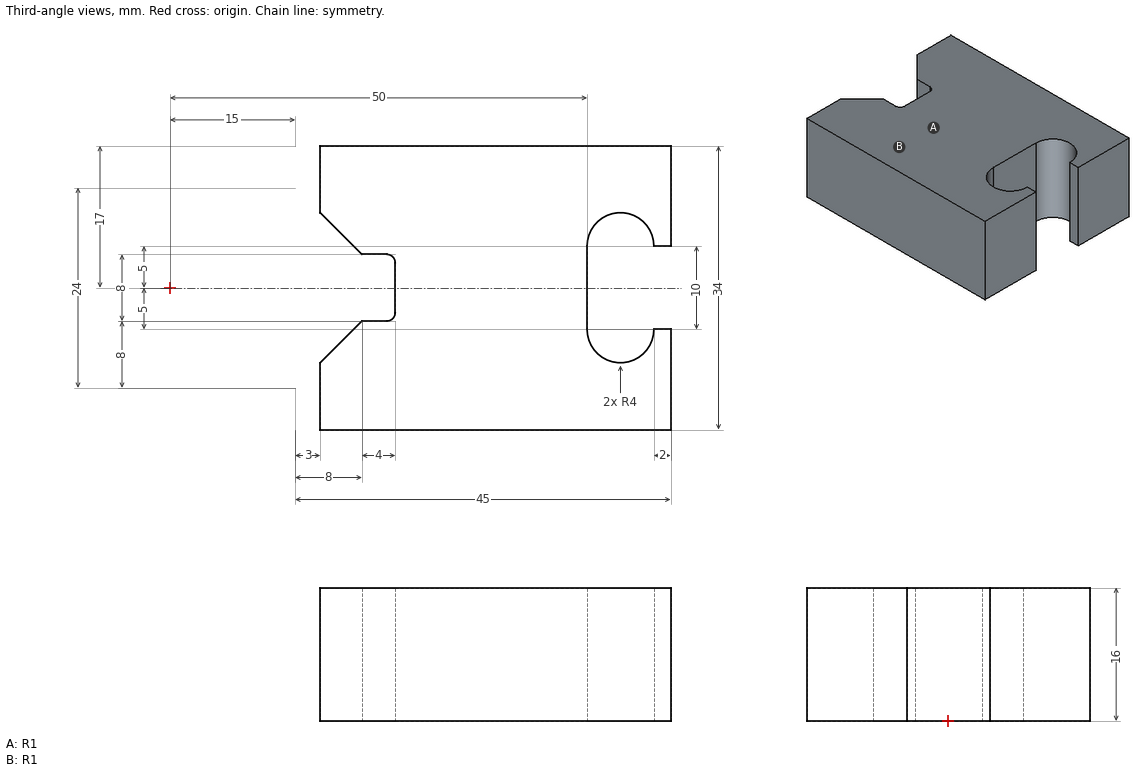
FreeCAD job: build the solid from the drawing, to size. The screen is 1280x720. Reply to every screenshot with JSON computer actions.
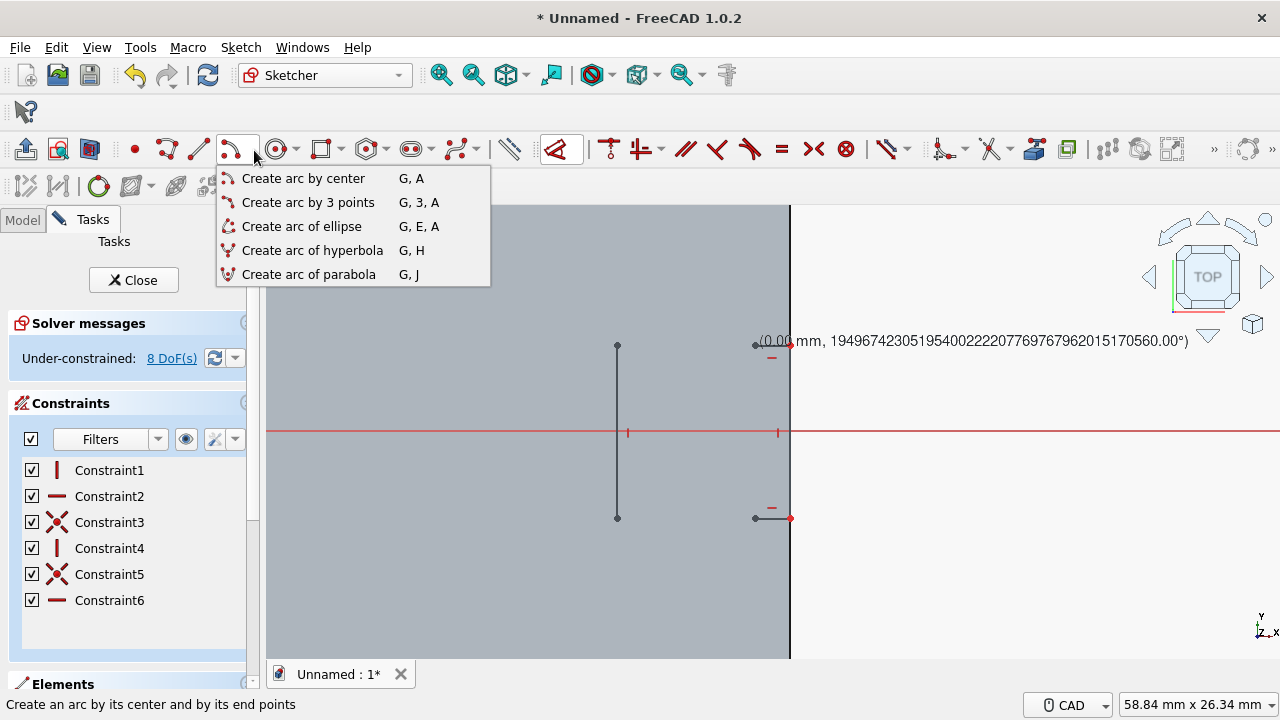
{"action": "left_click", "coordinate": [354, 202]}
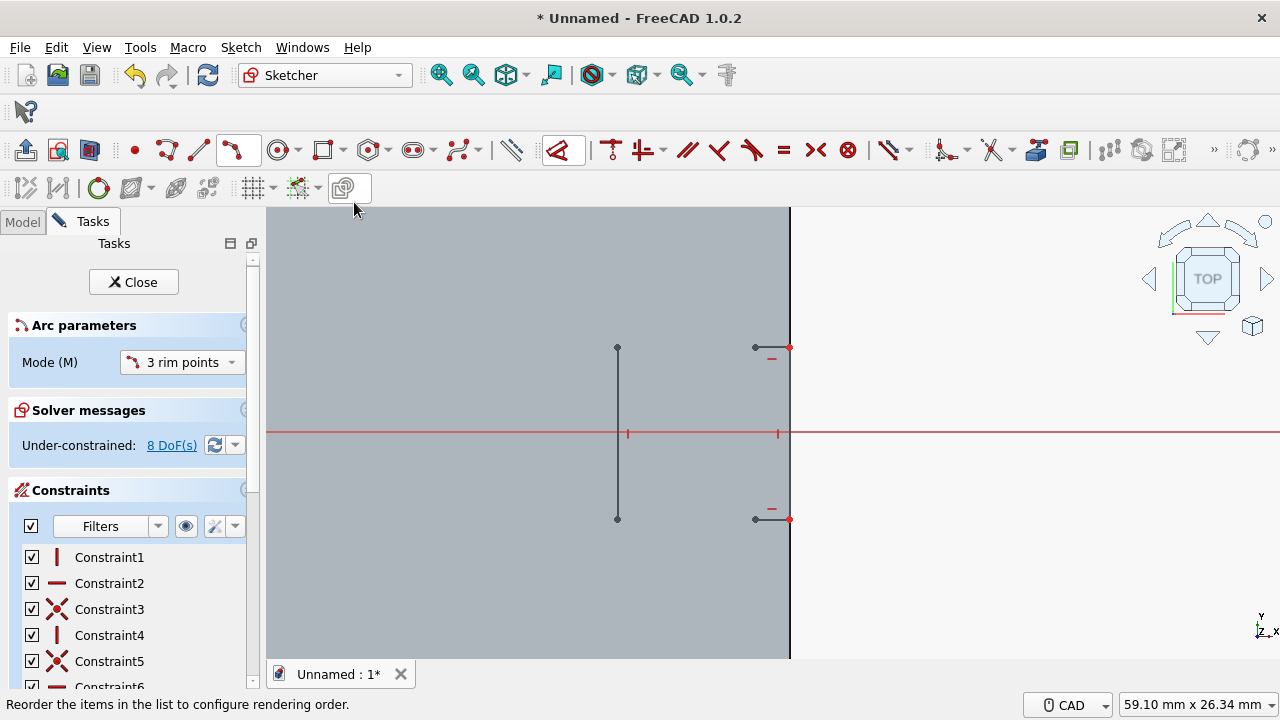
{"action": "left_click", "coordinate": [618, 520]}
{"action": "left_click", "coordinate": [755, 520]}
{"action": "left_click", "coordinate": [687, 587]}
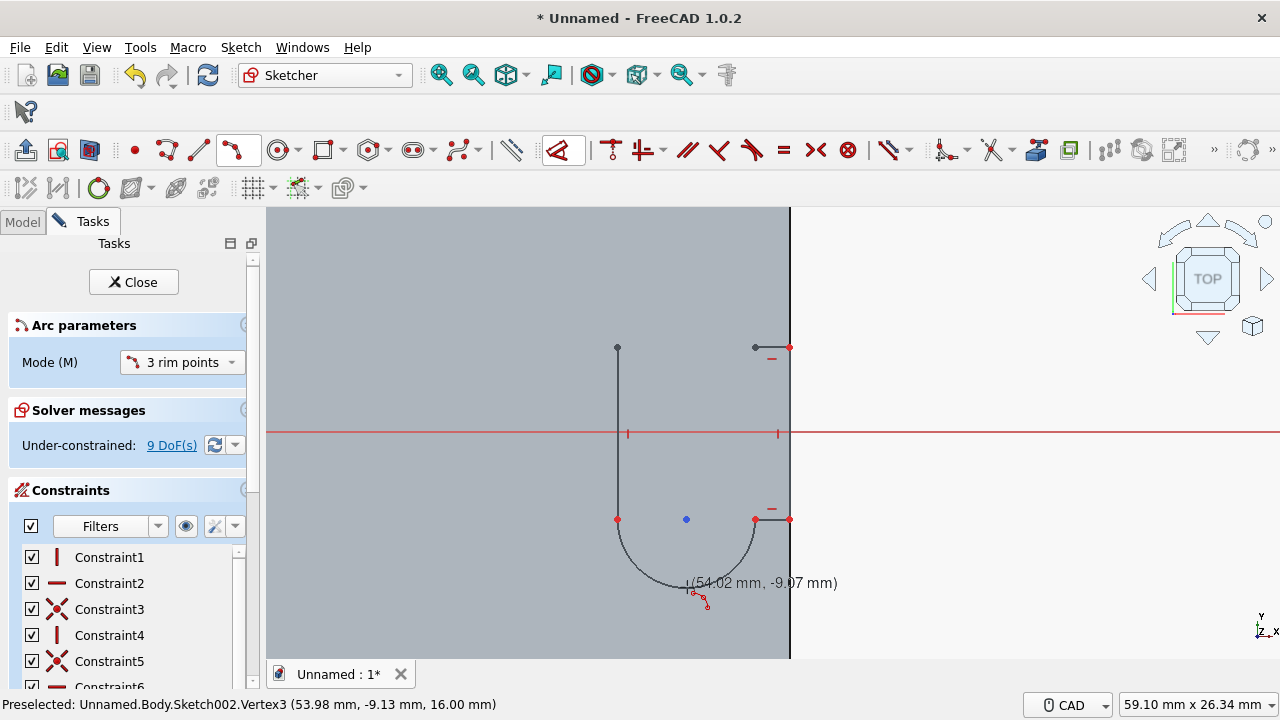
{"action": "left_click", "coordinate": [755, 347]}
{"action": "left_click", "coordinate": [618, 347]}
{"action": "left_click", "coordinate": [687, 278]}
{"action": "key", "text": "Escape"}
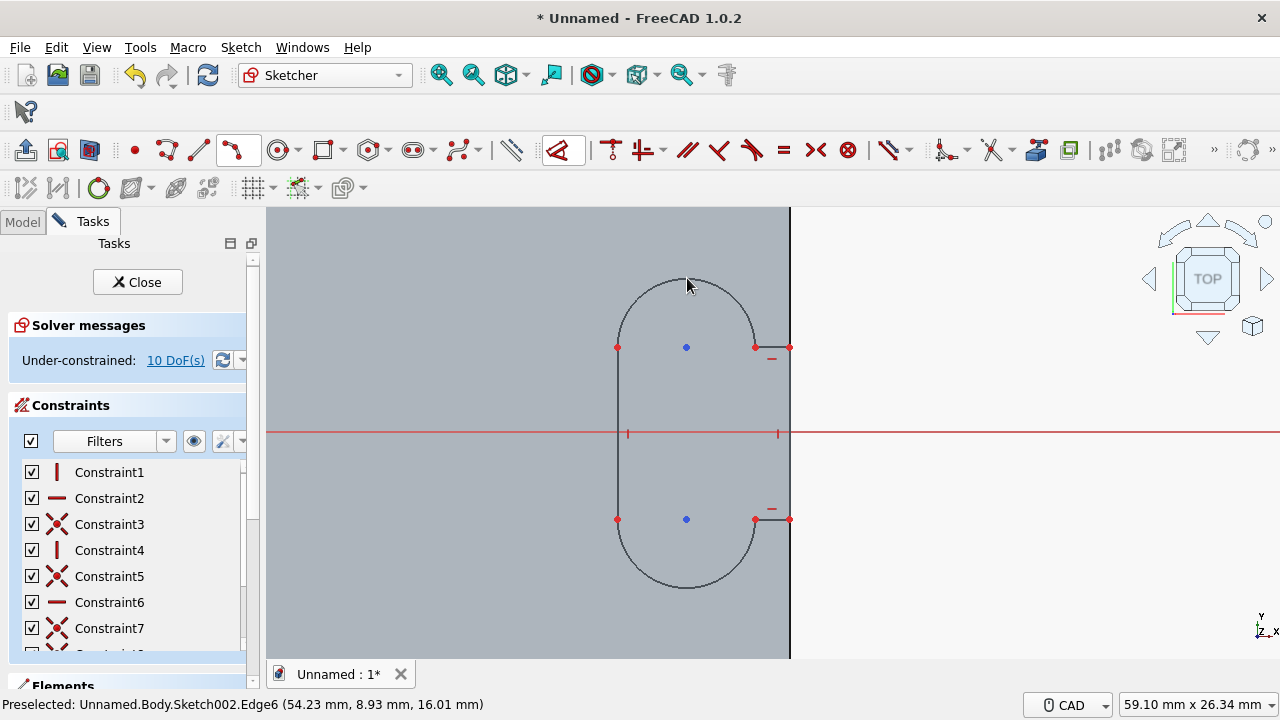
{"action": "left_click", "coordinate": [618, 399]}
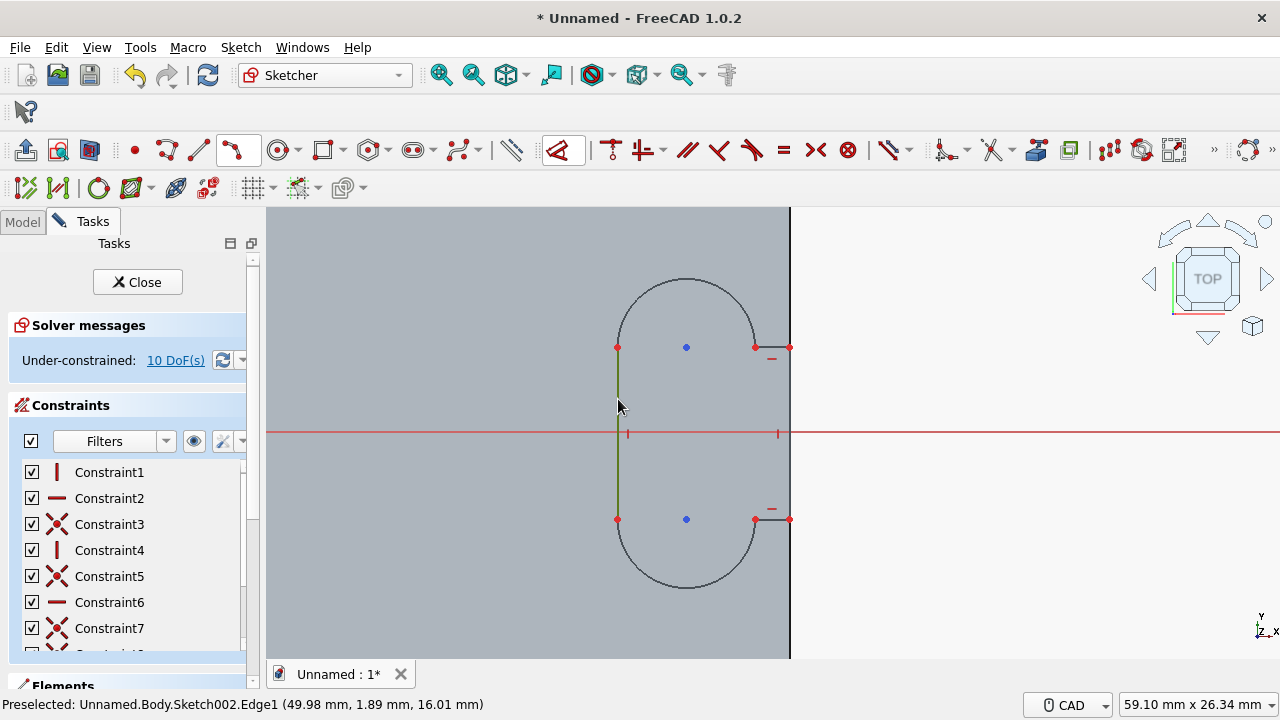
{"action": "left_click", "coordinate": [646, 575]}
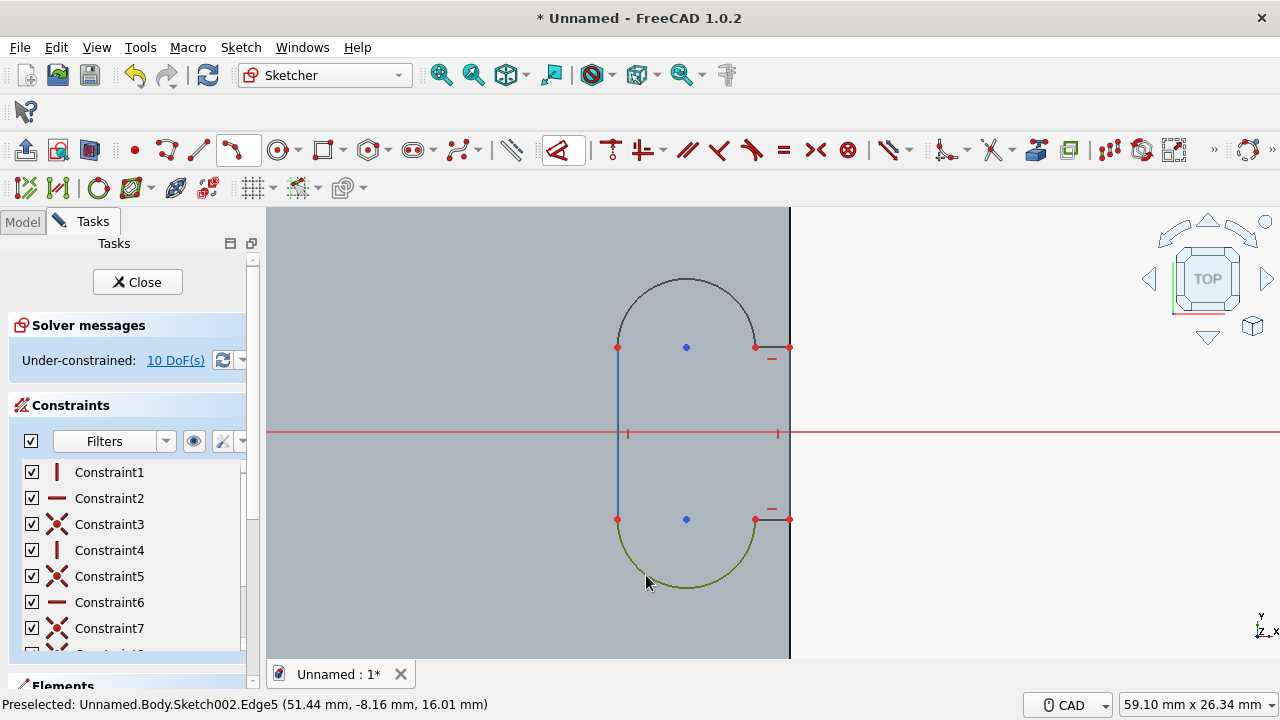
{"action": "left_click", "coordinate": [752, 150]}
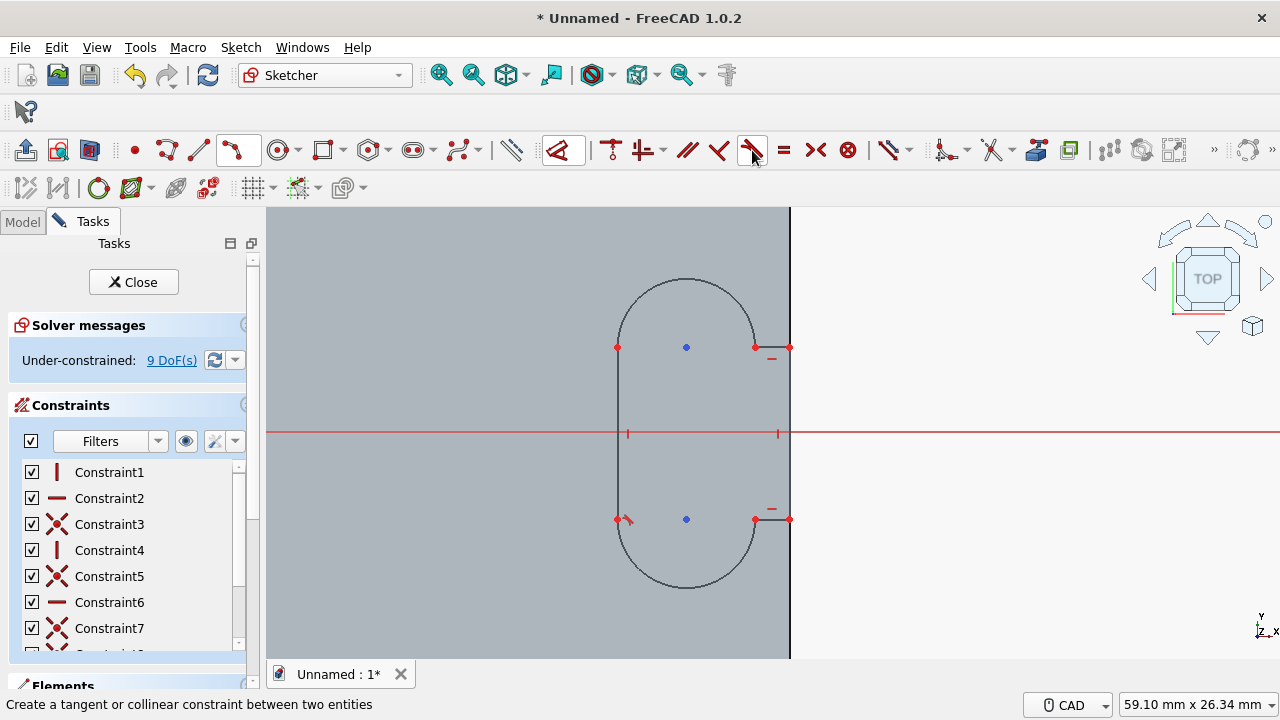
{"action": "left_click", "coordinate": [618, 399]}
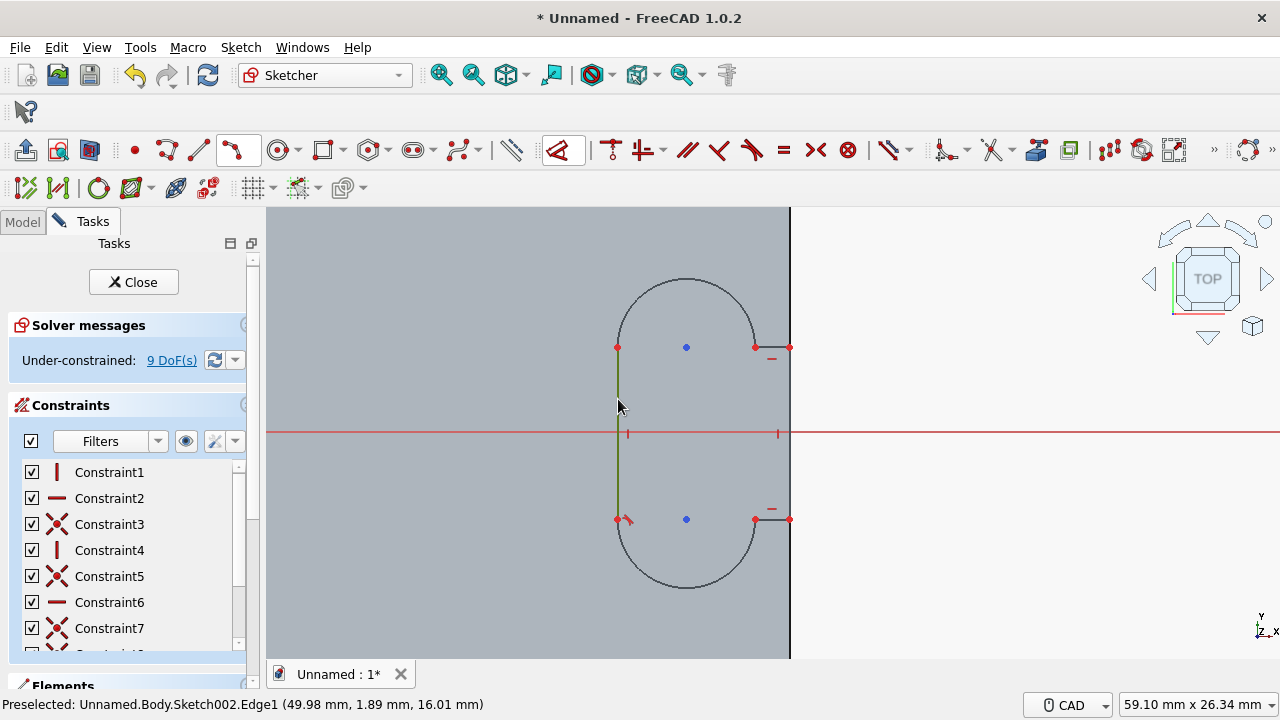
{"action": "left_click", "coordinate": [727, 292]}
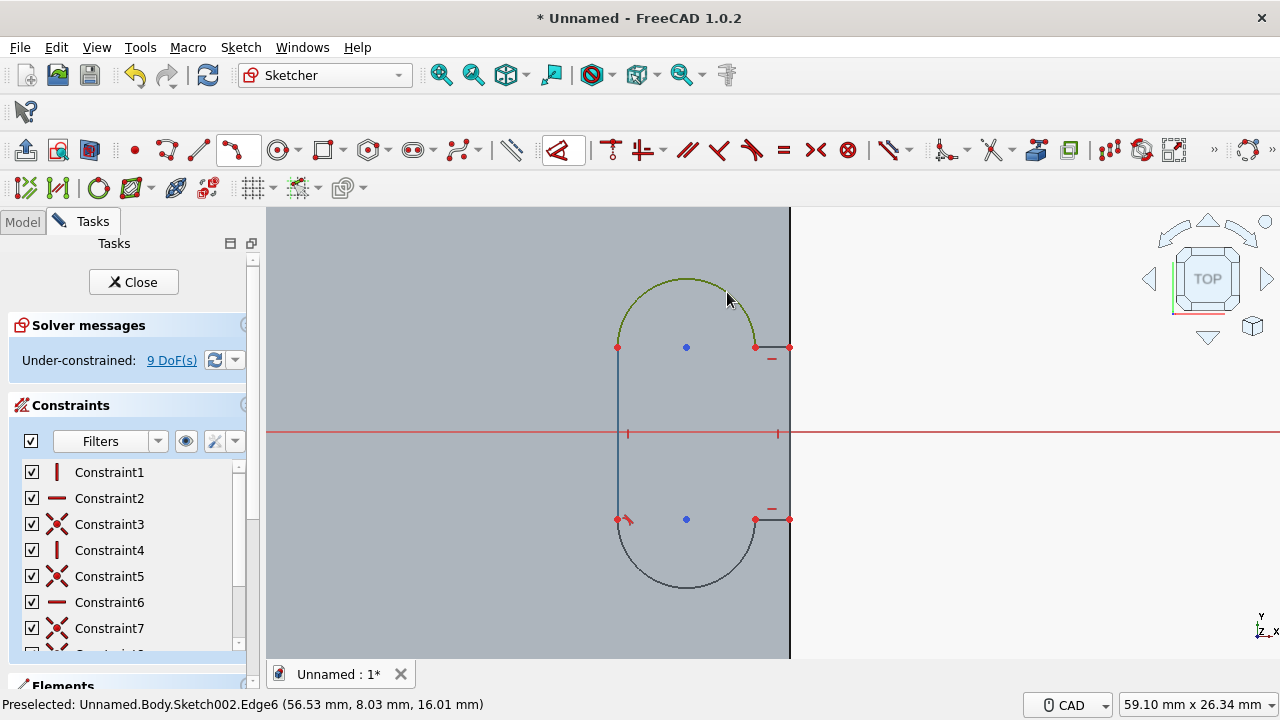
{"action": "left_click", "coordinate": [752, 150]}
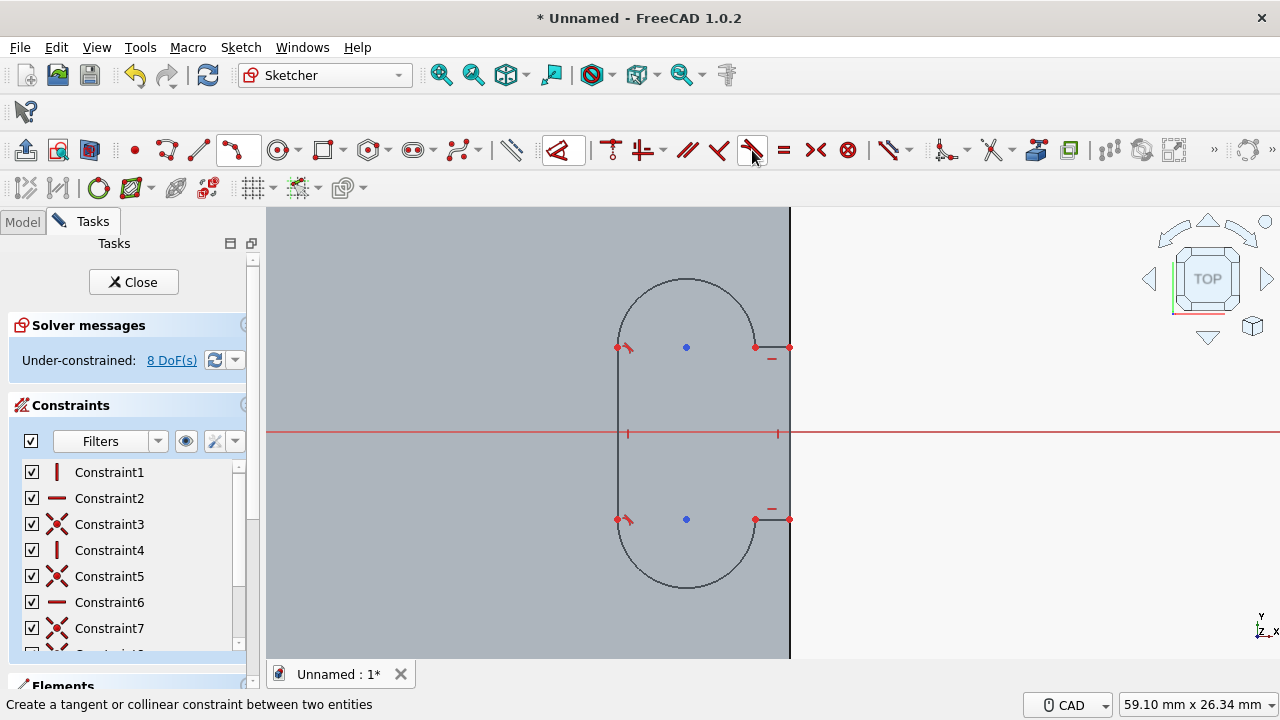
{"action": "left_click", "coordinate": [646, 575]}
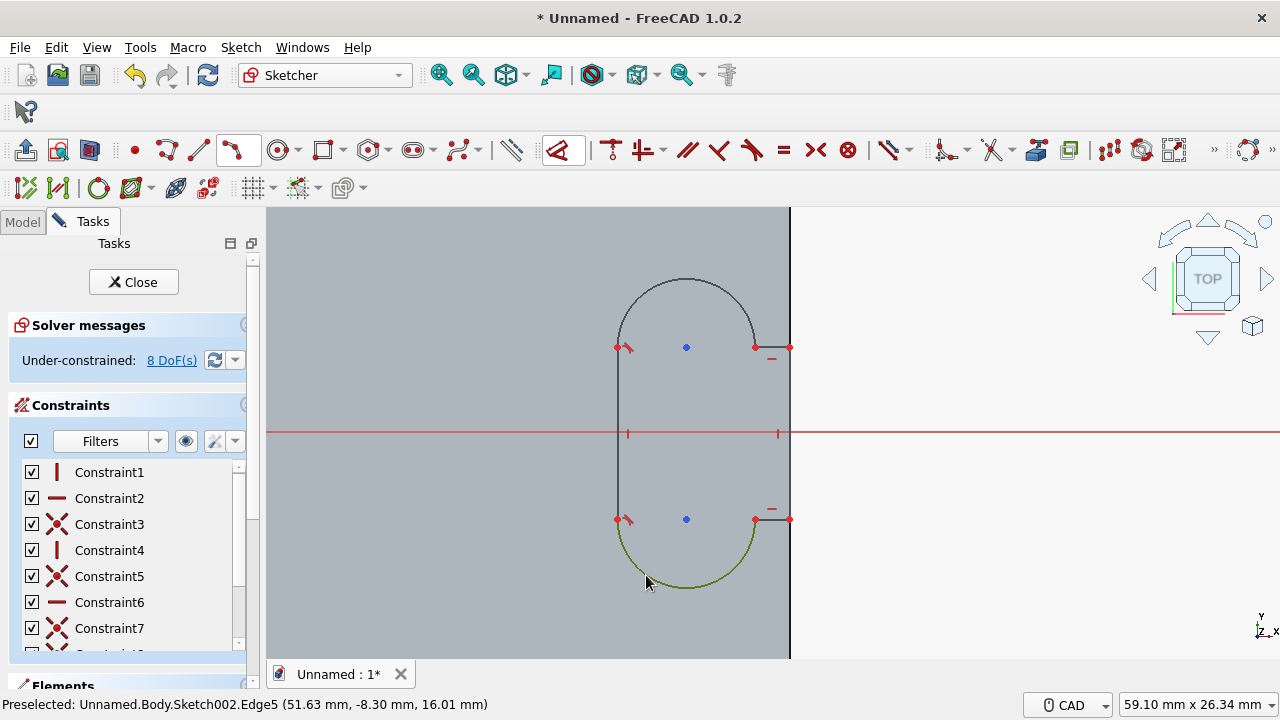
{"action": "left_click", "coordinate": [727, 292]}